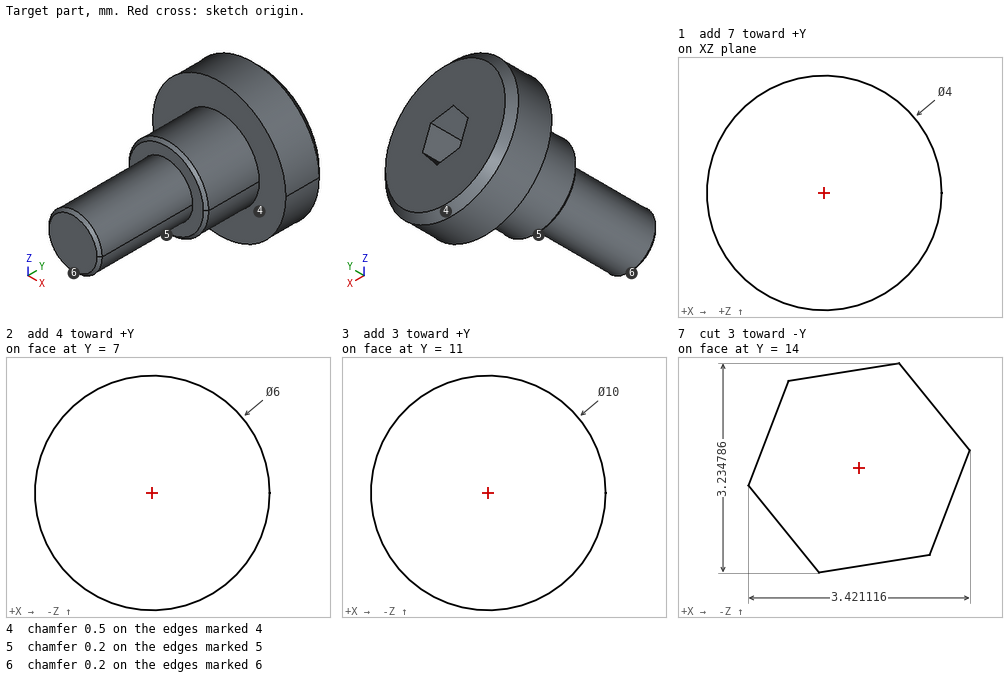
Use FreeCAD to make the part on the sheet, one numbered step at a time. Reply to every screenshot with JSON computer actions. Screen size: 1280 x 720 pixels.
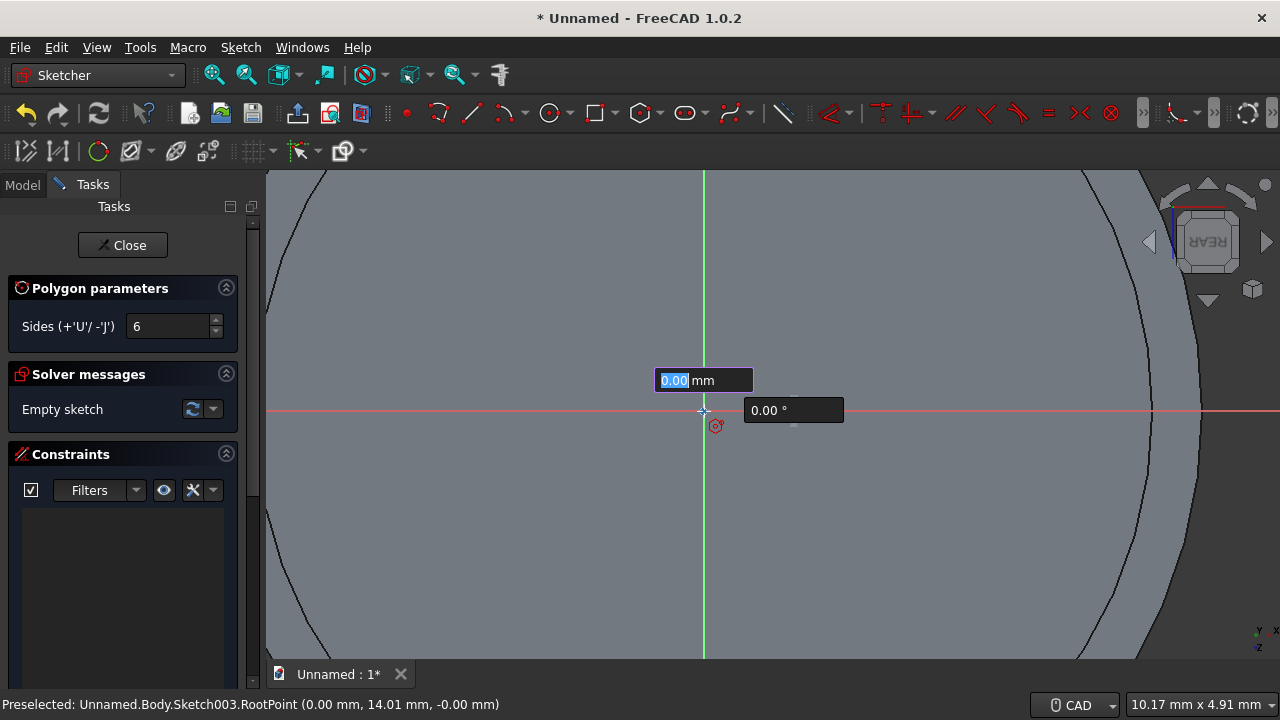
{"action": "left_click", "coordinate": [812, 546]}
{"action": "right_click", "coordinate": [812, 546]}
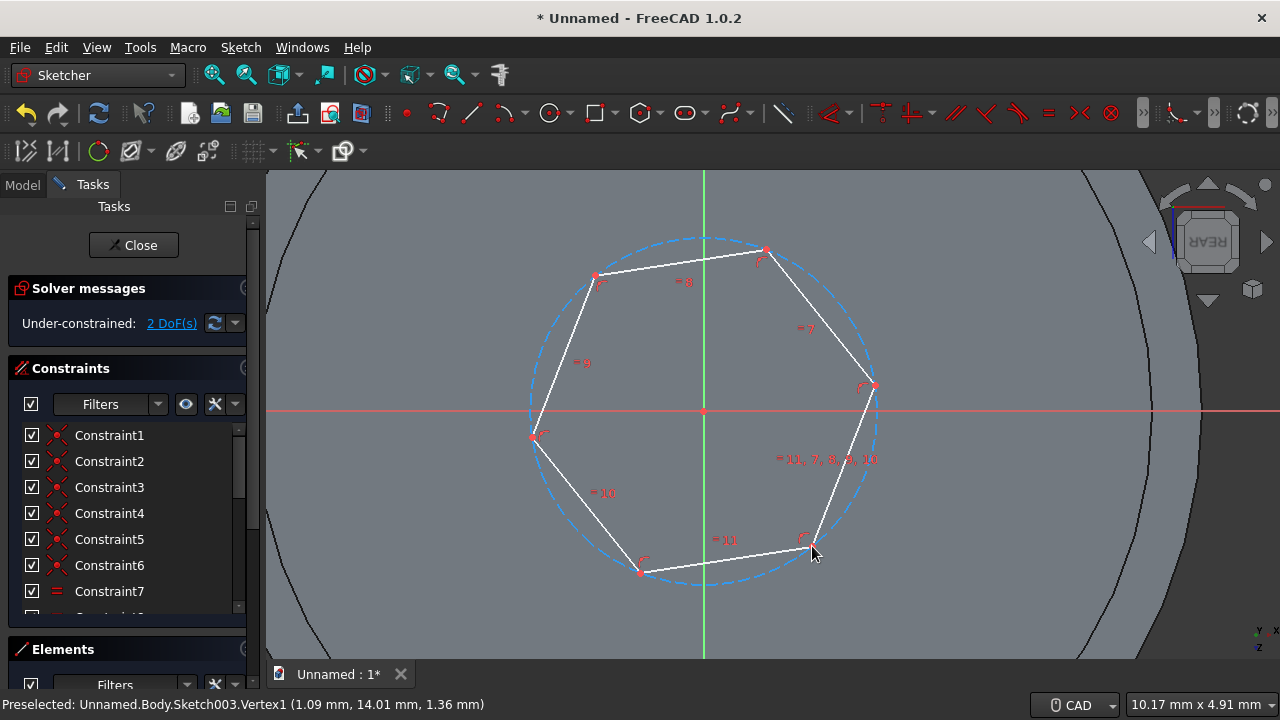
{"action": "left_click", "coordinate": [830, 114]}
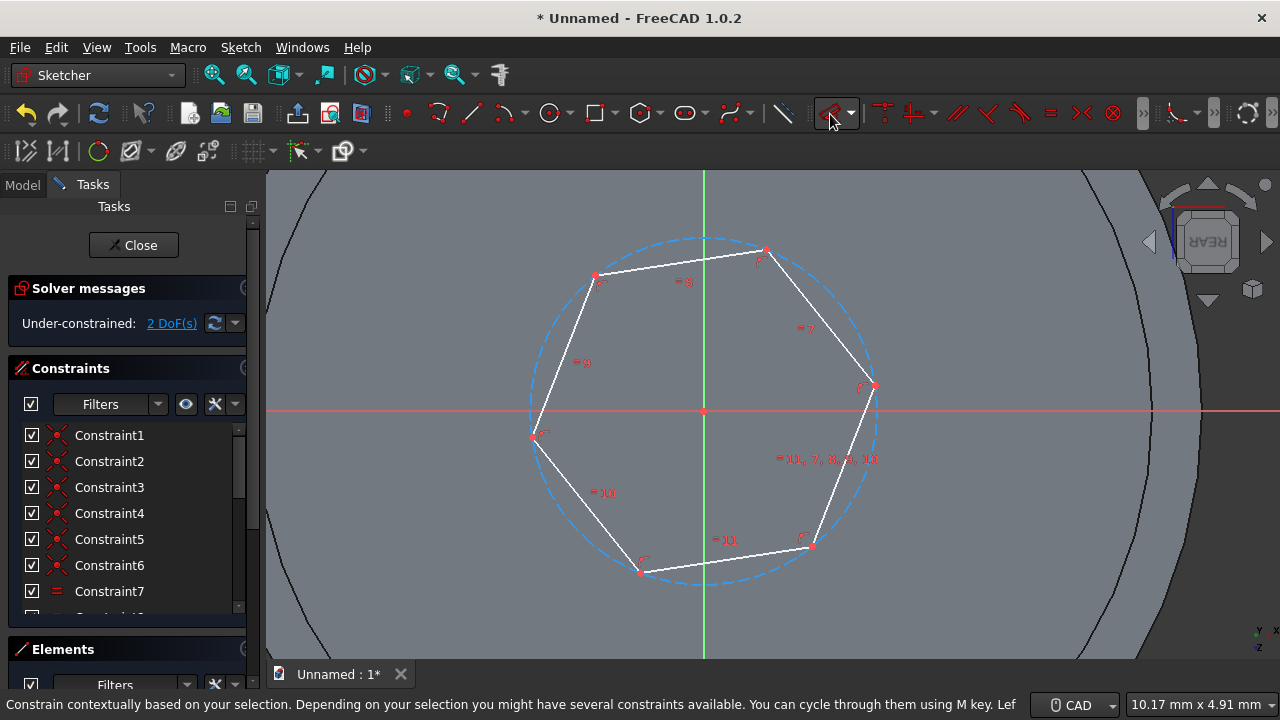
{"action": "left_click", "coordinate": [532, 438]}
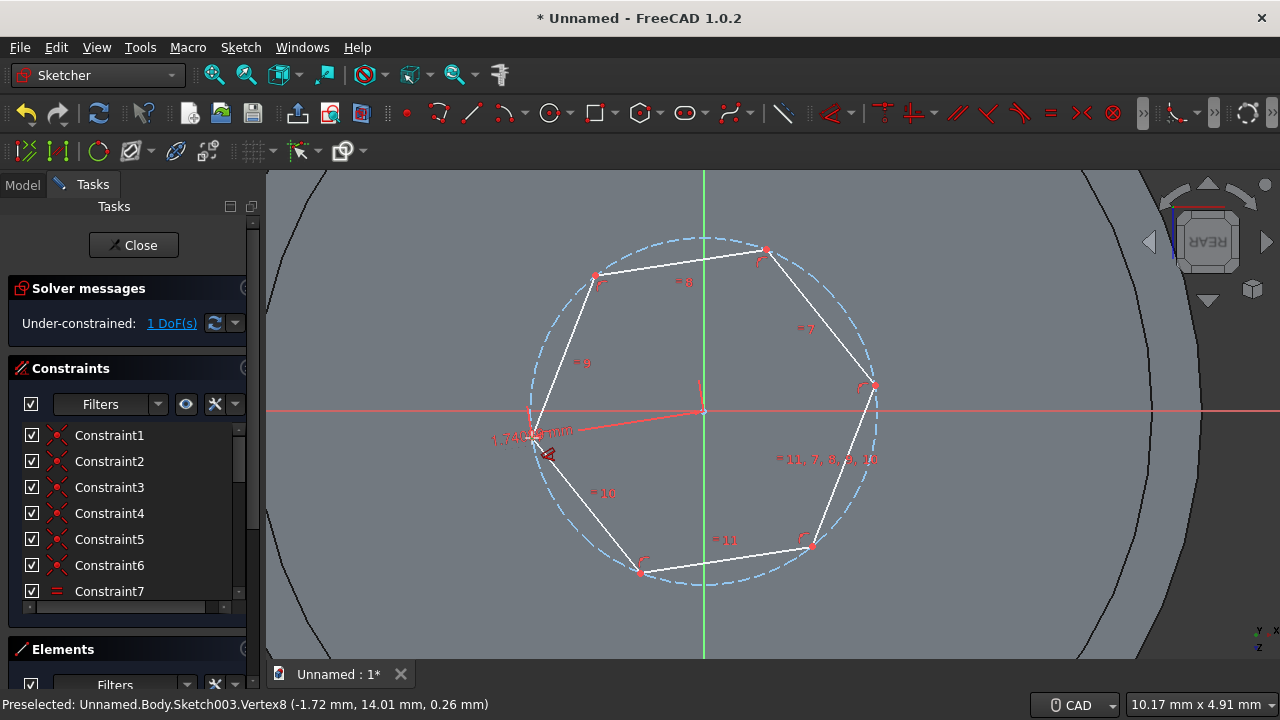
{"action": "left_click", "coordinate": [875, 385]}
{"action": "left_click", "coordinate": [625, 351]}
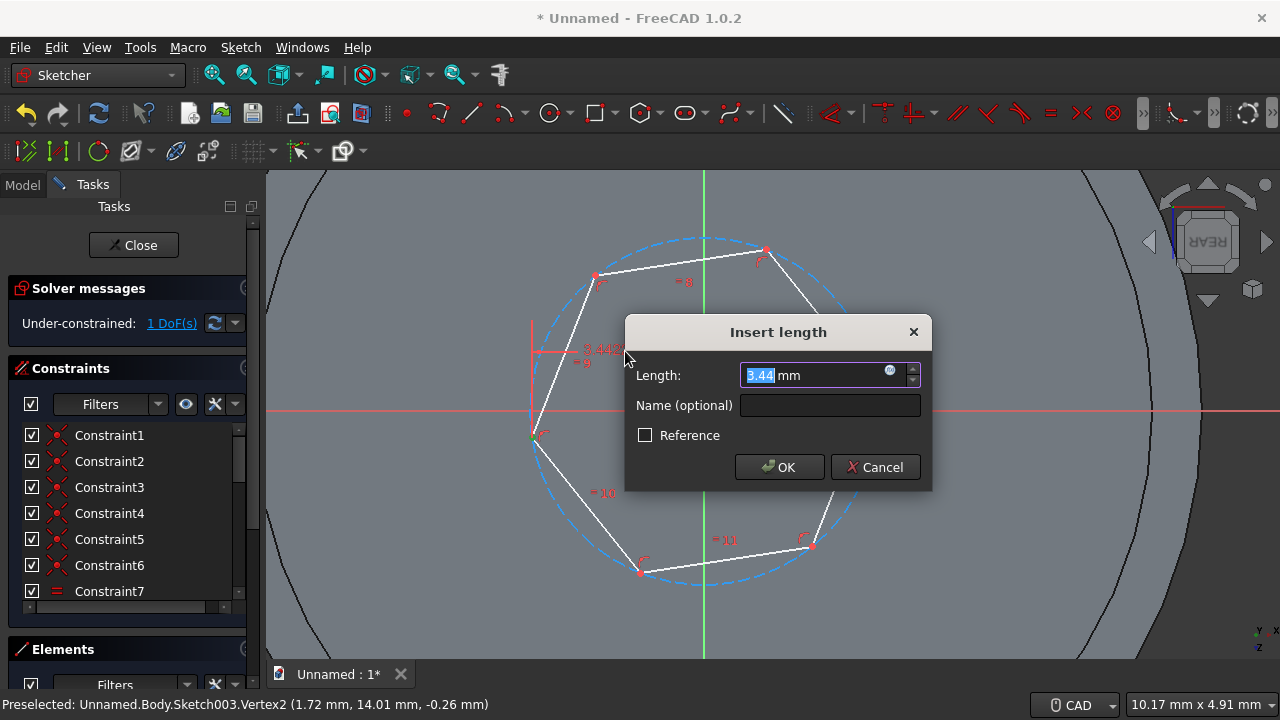
{"action": "type", "text": "3.421116"}
{"action": "key", "text": "Return"}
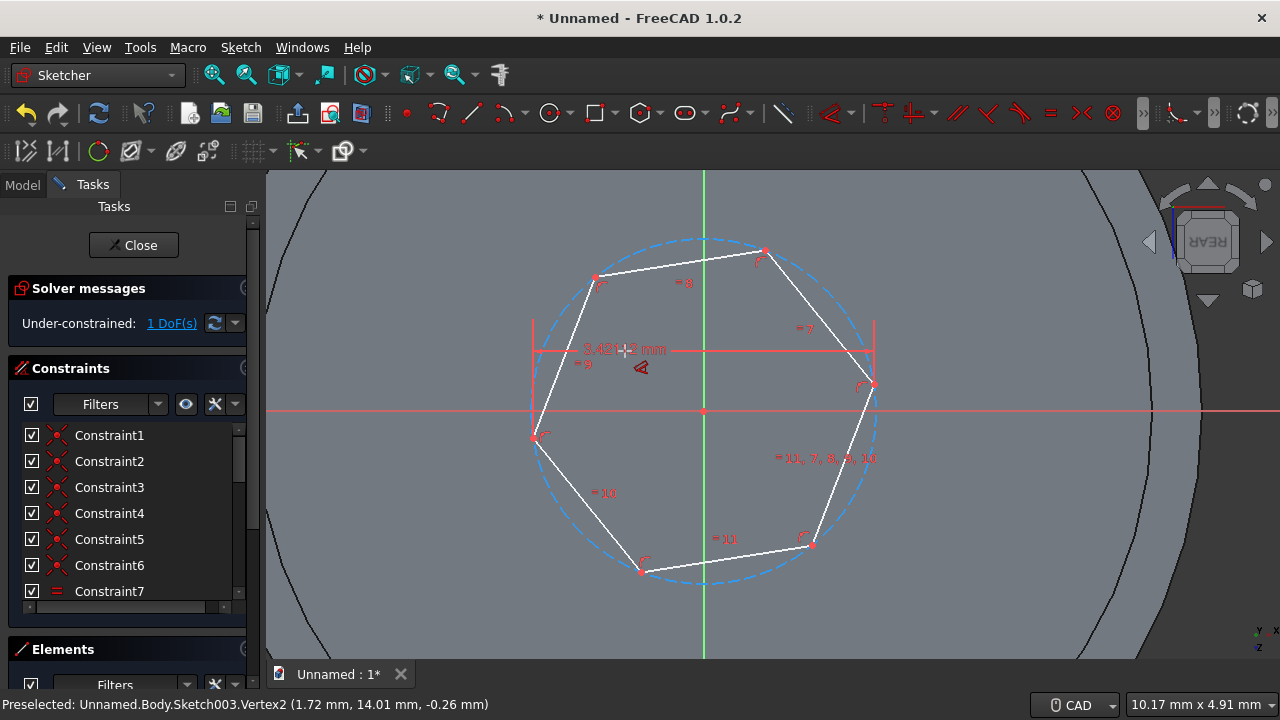
{"action": "left_click", "coordinate": [641, 572]}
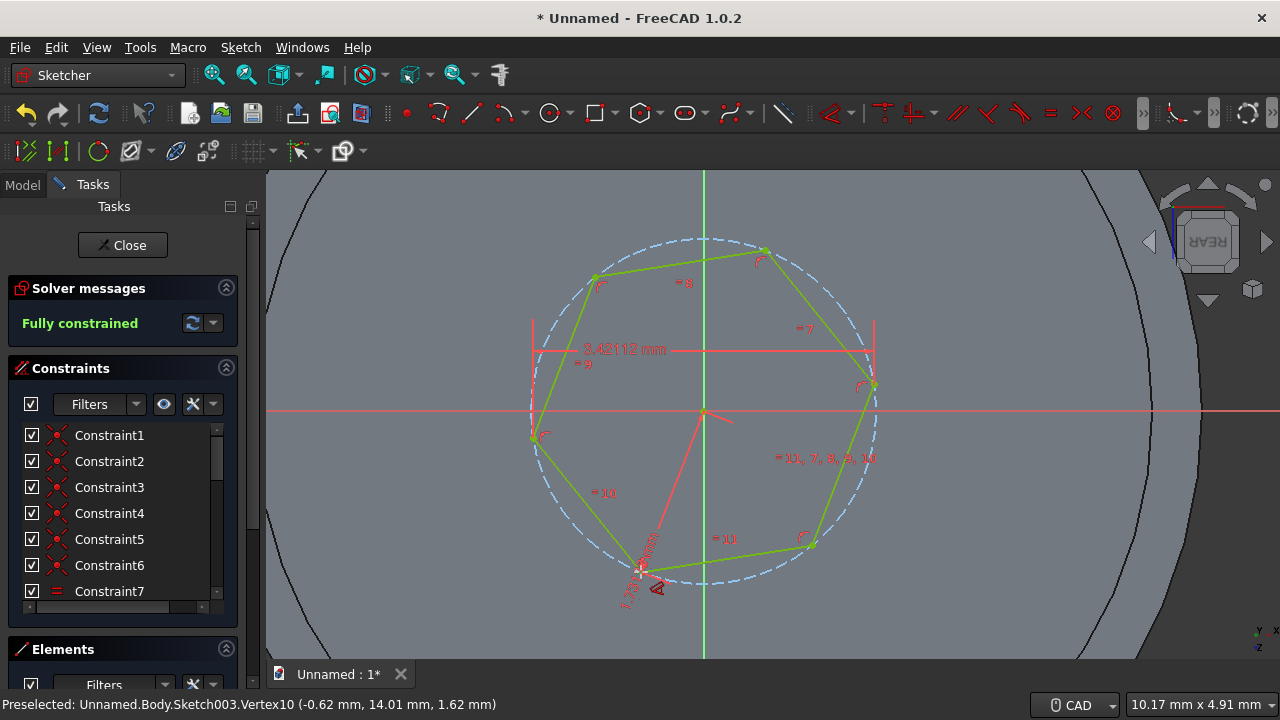
{"action": "left_click", "coordinate": [766, 250]}
{"action": "left_click", "coordinate": [800, 337]}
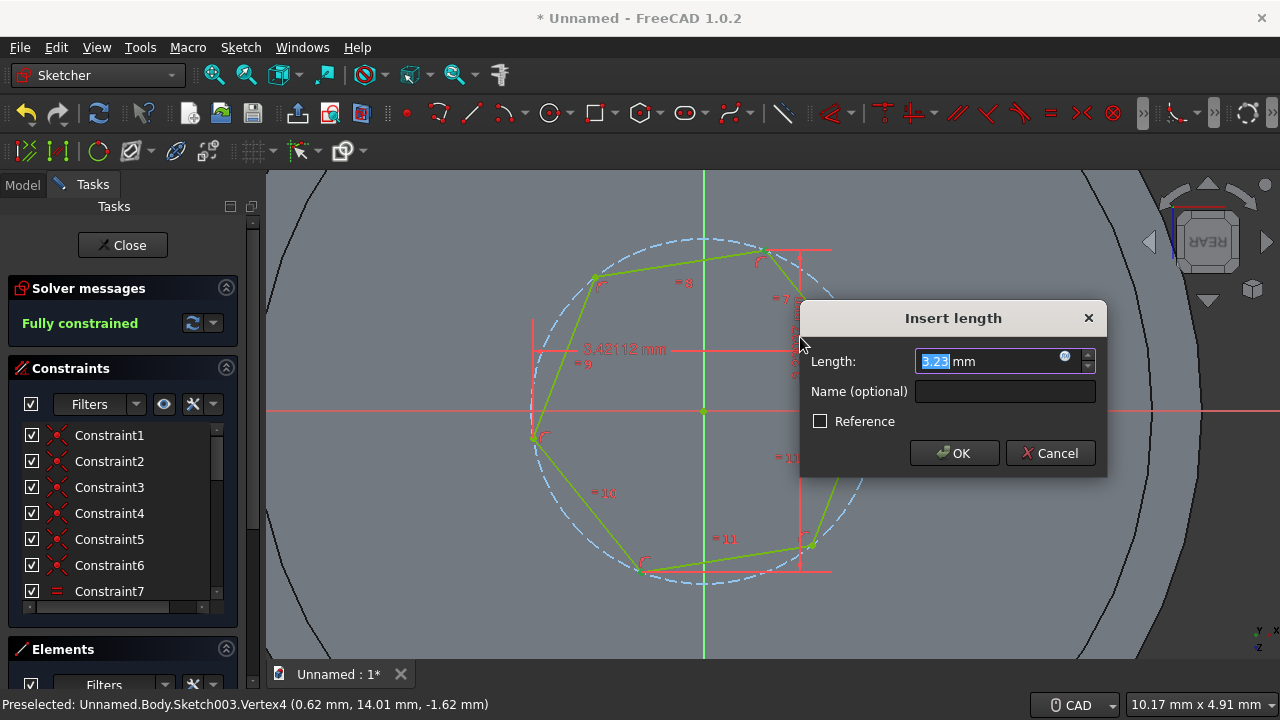
{"action": "type", "text": "3.234786"}
{"action": "key", "text": "Return"}
{"action": "key", "text": "Escape"}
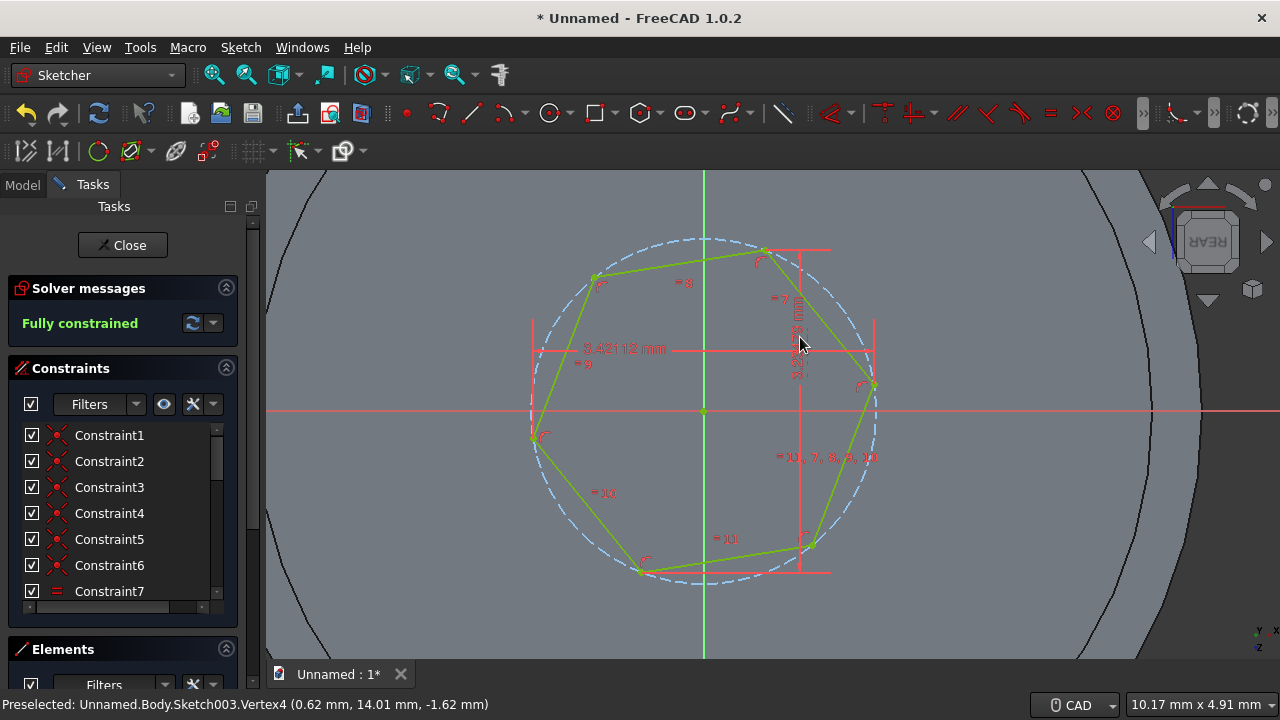
{"action": "left_click", "coordinate": [123, 245]}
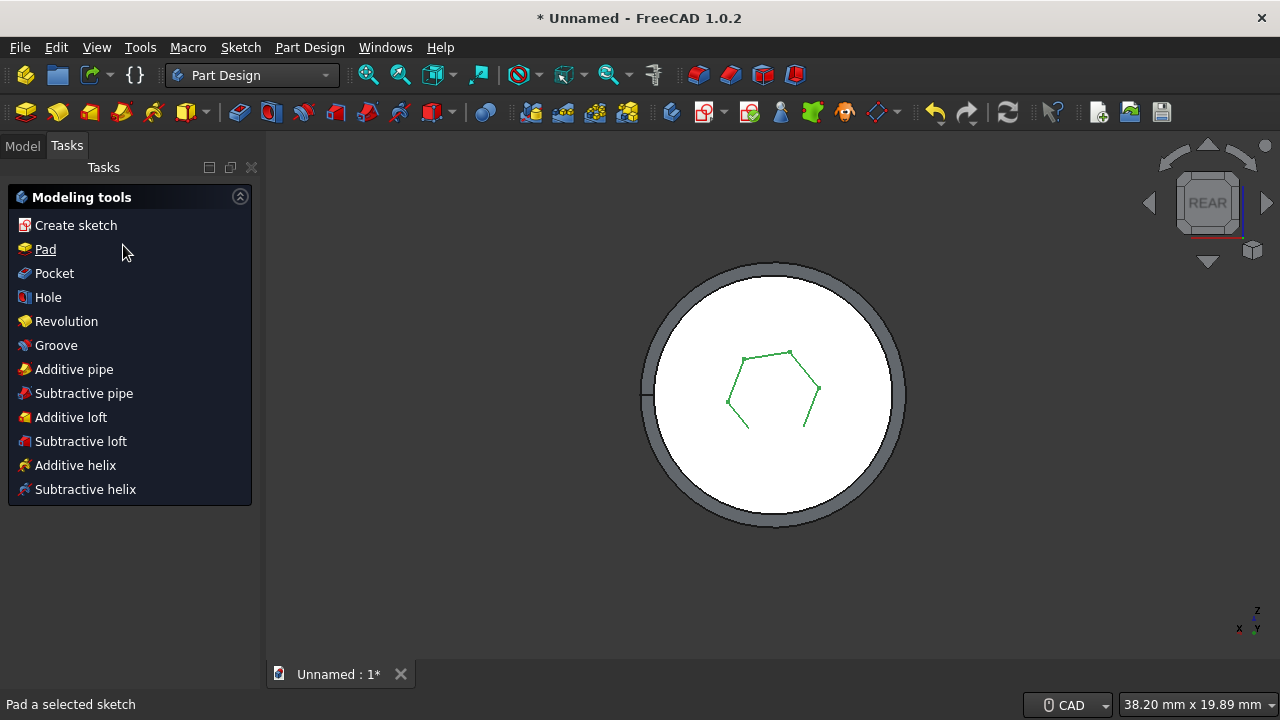
{"action": "left_click", "coordinate": [240, 112]}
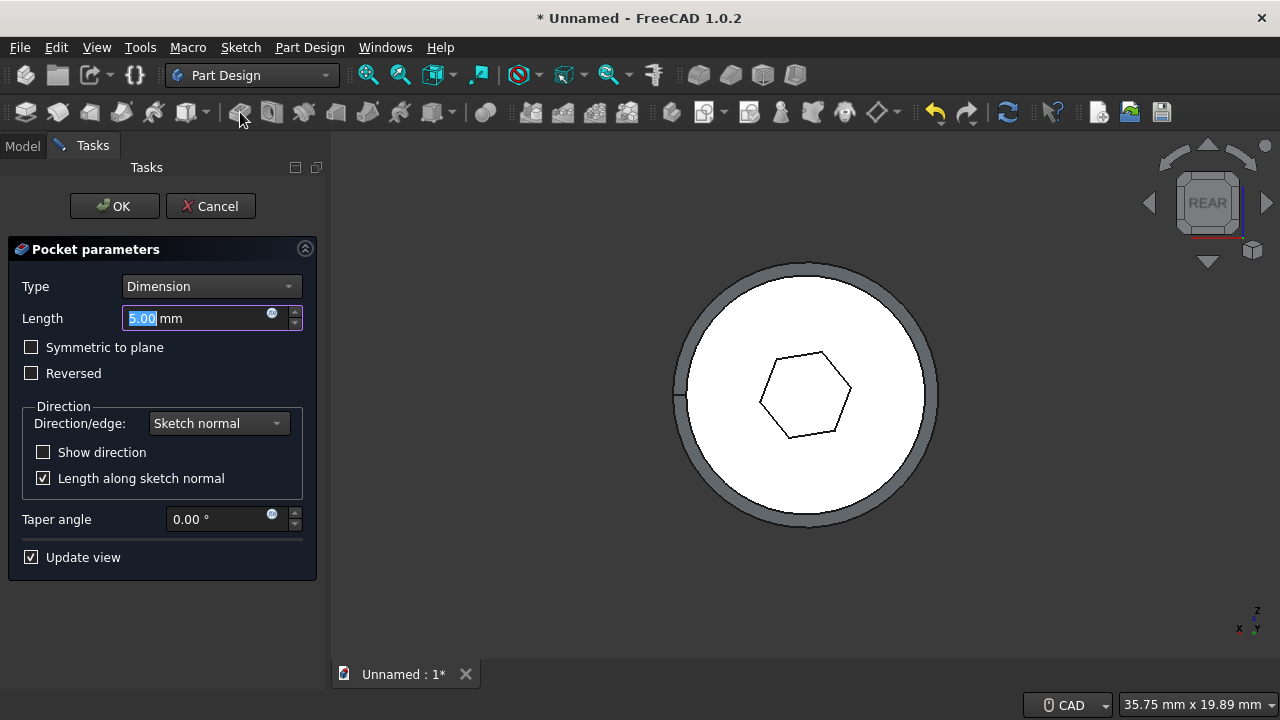
{"action": "type", "text": "3"}
{"action": "key", "text": "Tab"}